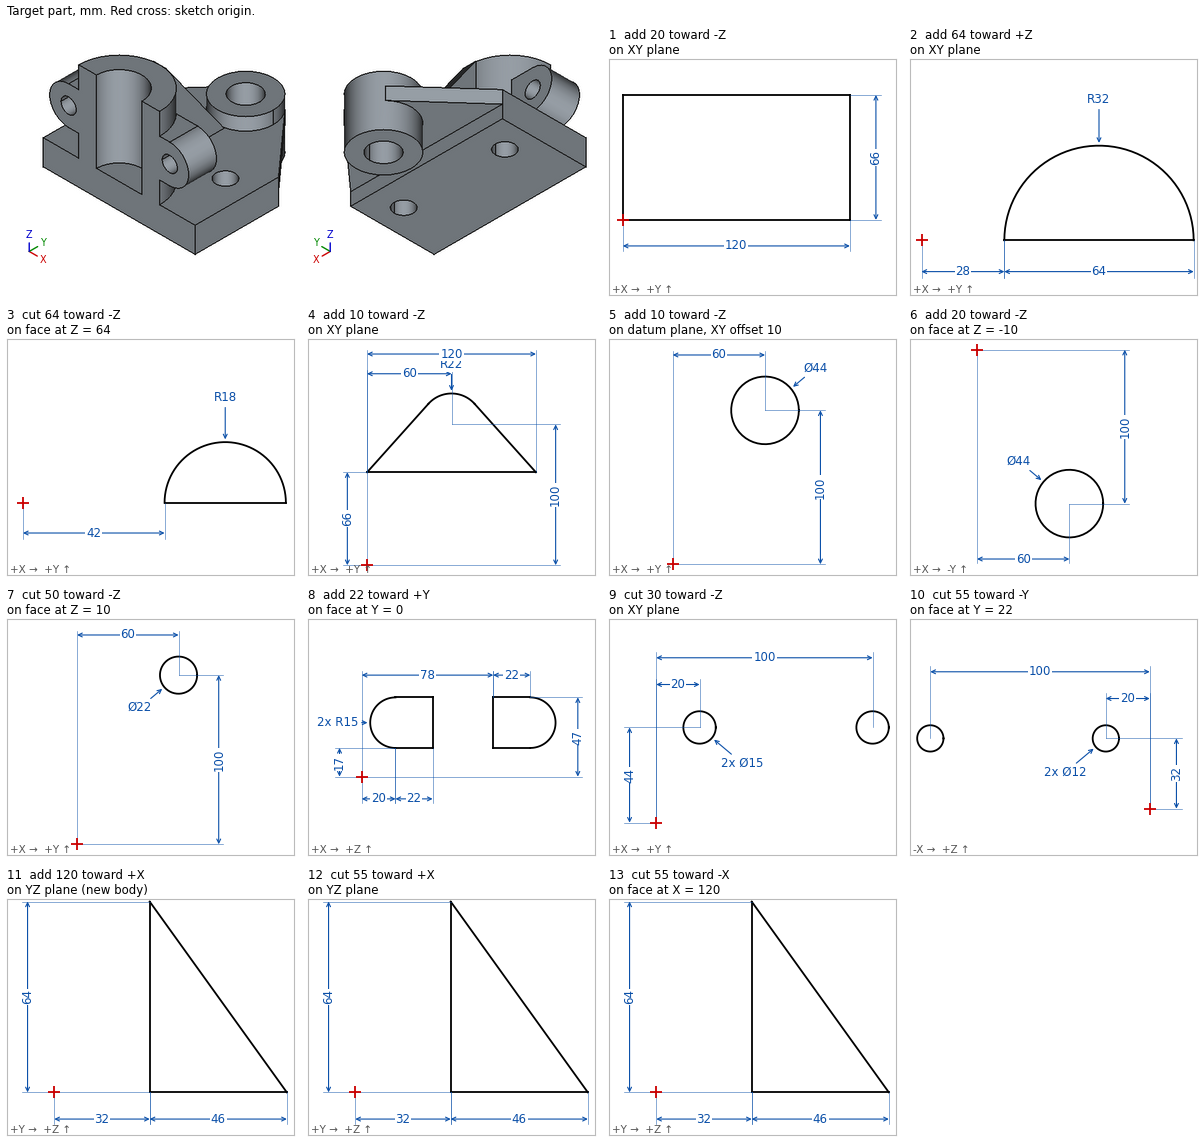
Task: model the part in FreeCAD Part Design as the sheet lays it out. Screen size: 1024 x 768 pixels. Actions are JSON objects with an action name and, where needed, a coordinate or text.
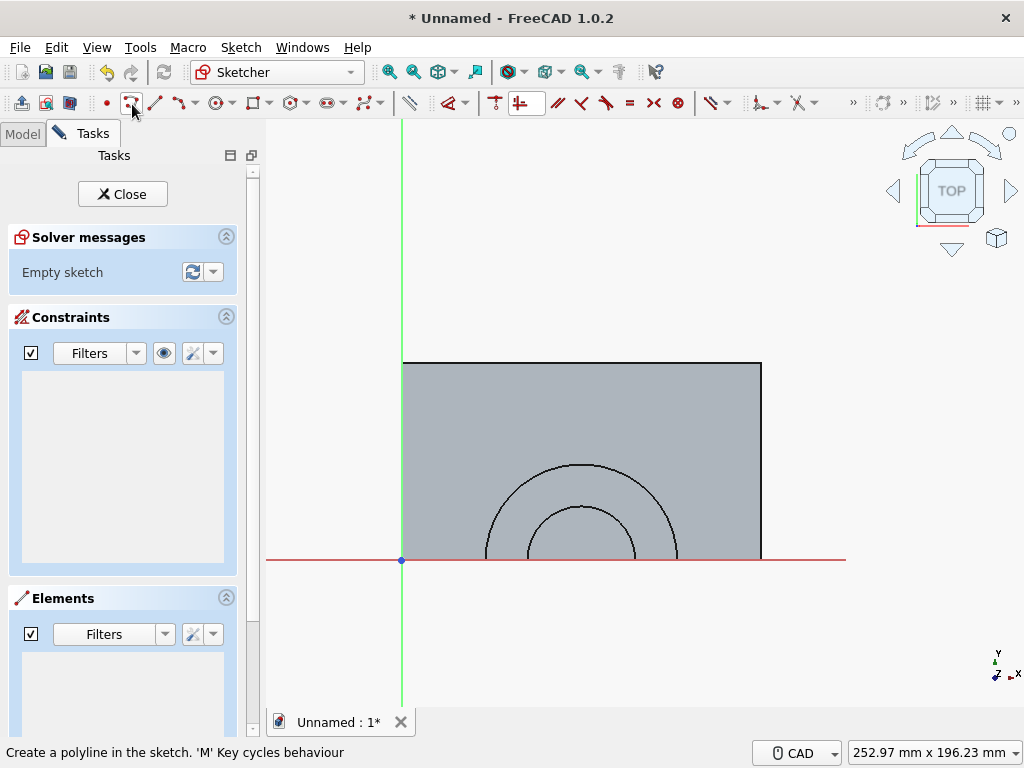
{"action": "left_click", "coordinate": [532, 217]}
{"action": "left_click", "coordinate": [402, 363]}
{"action": "left_click", "coordinate": [761, 363]}
{"action": "left_click", "coordinate": [630, 217]}
{"action": "right_click", "coordinate": [630, 217]}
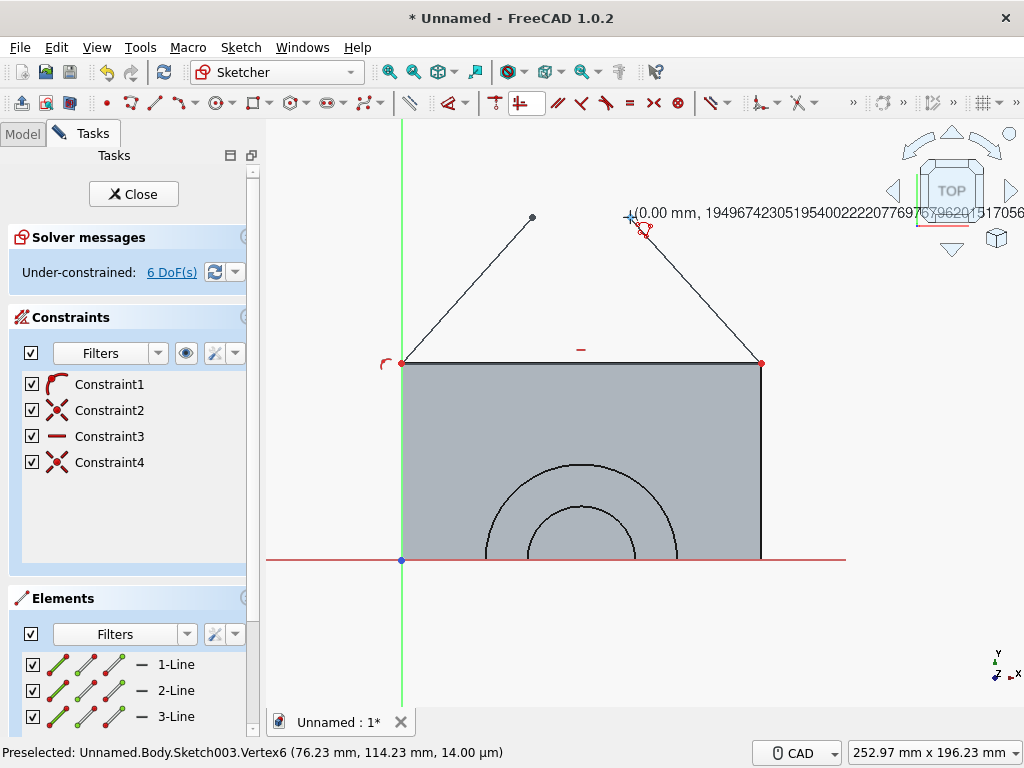
{"action": "left_click", "coordinate": [180, 104]}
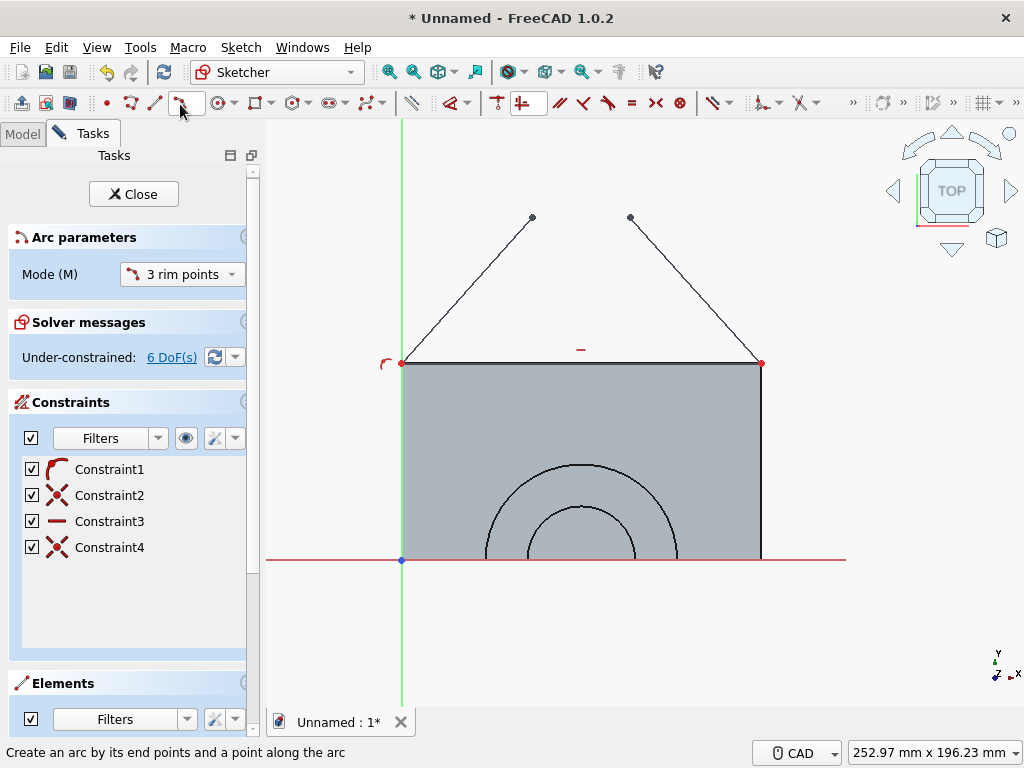
{"action": "left_click", "coordinate": [630, 218]}
{"action": "left_click", "coordinate": [532, 218]}
{"action": "left_click", "coordinate": [581, 195]}
{"action": "key", "text": "Escape"}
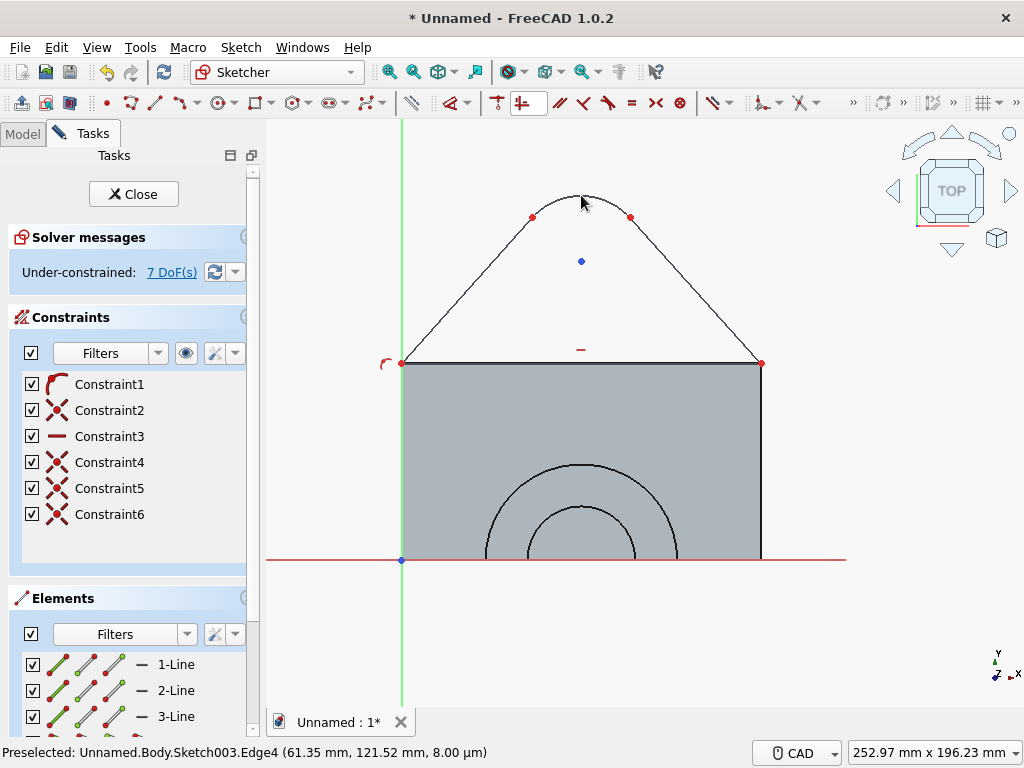
{"action": "left_click", "coordinate": [493, 262]}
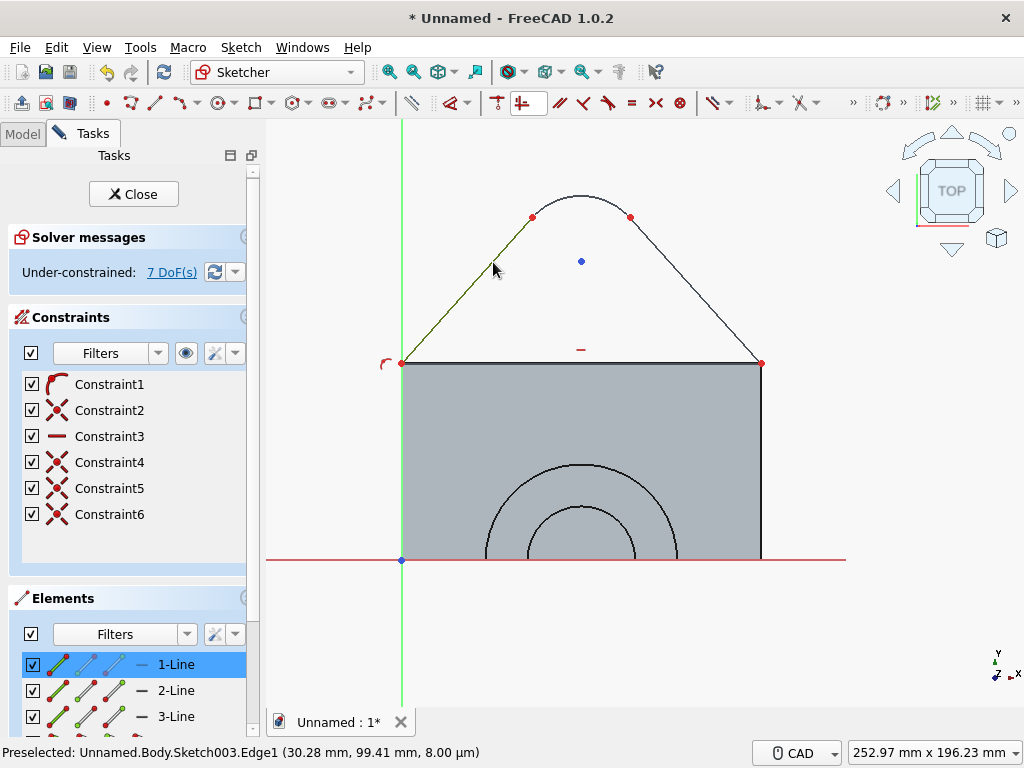
{"action": "left_click", "coordinate": [603, 200]}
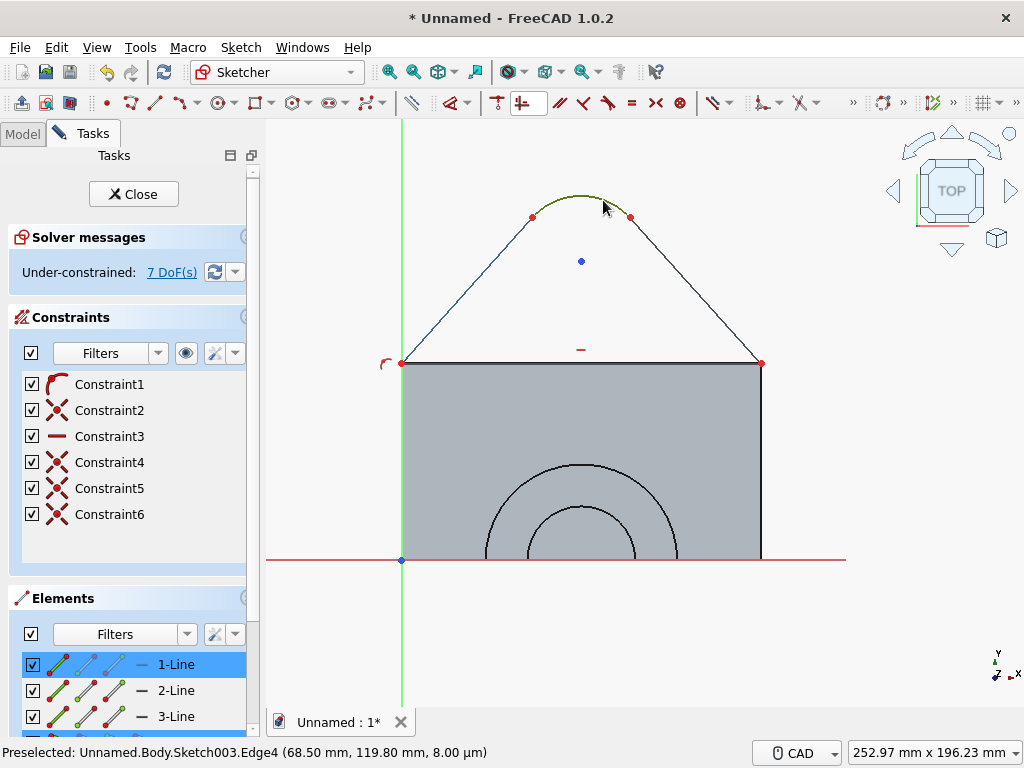
{"action": "left_click", "coordinate": [608, 104]}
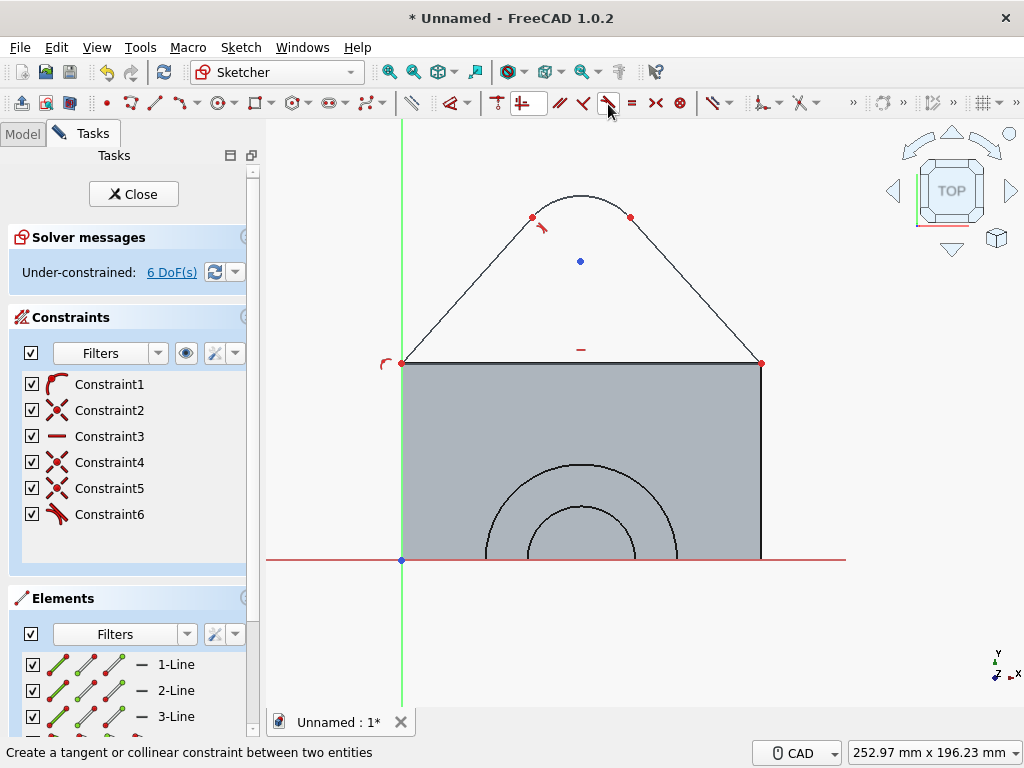
{"action": "left_click", "coordinate": [722, 320]}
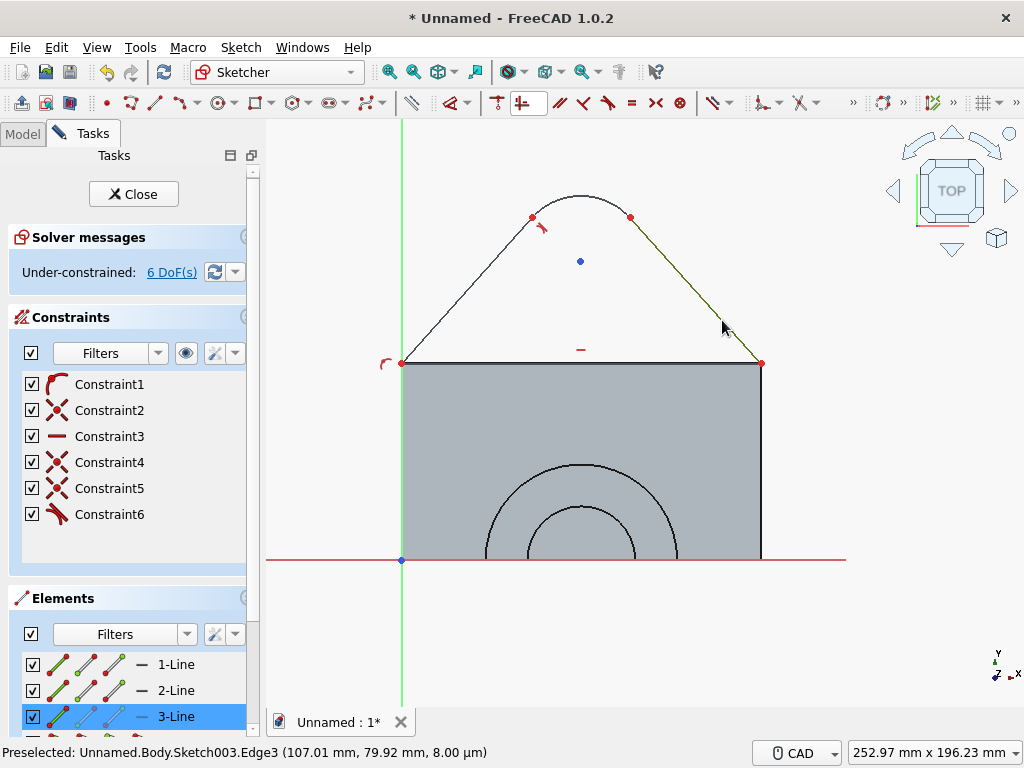
{"action": "left_click", "coordinate": [603, 200]}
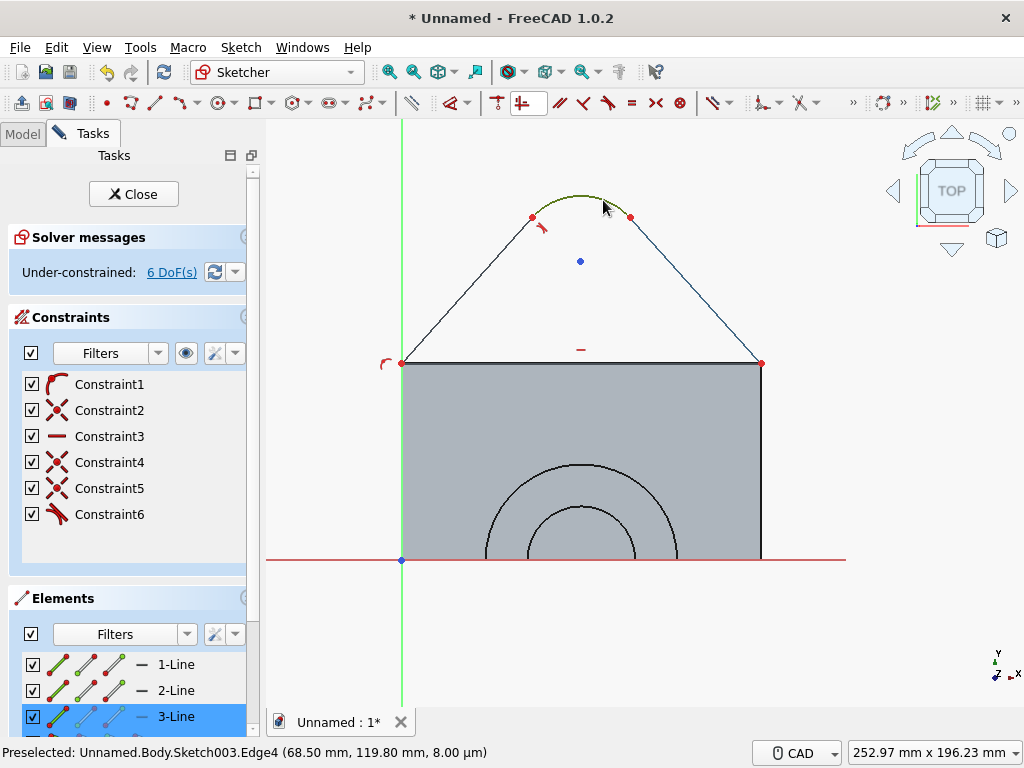
{"action": "left_click", "coordinate": [608, 104]}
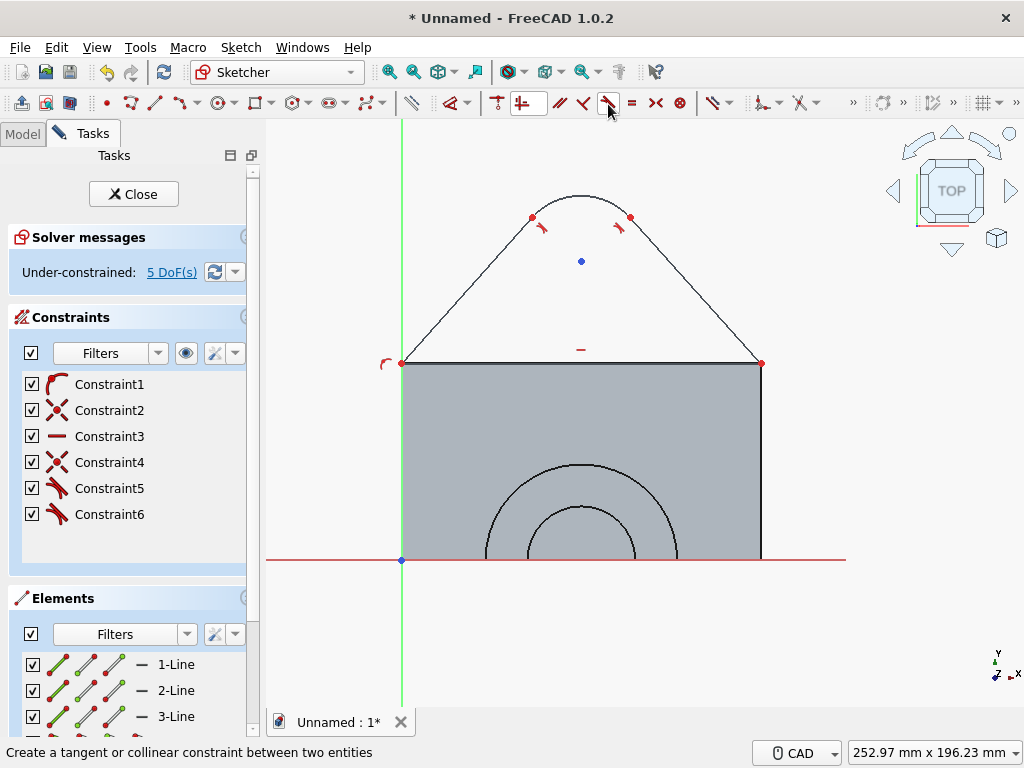
{"action": "left_click", "coordinate": [450, 104]}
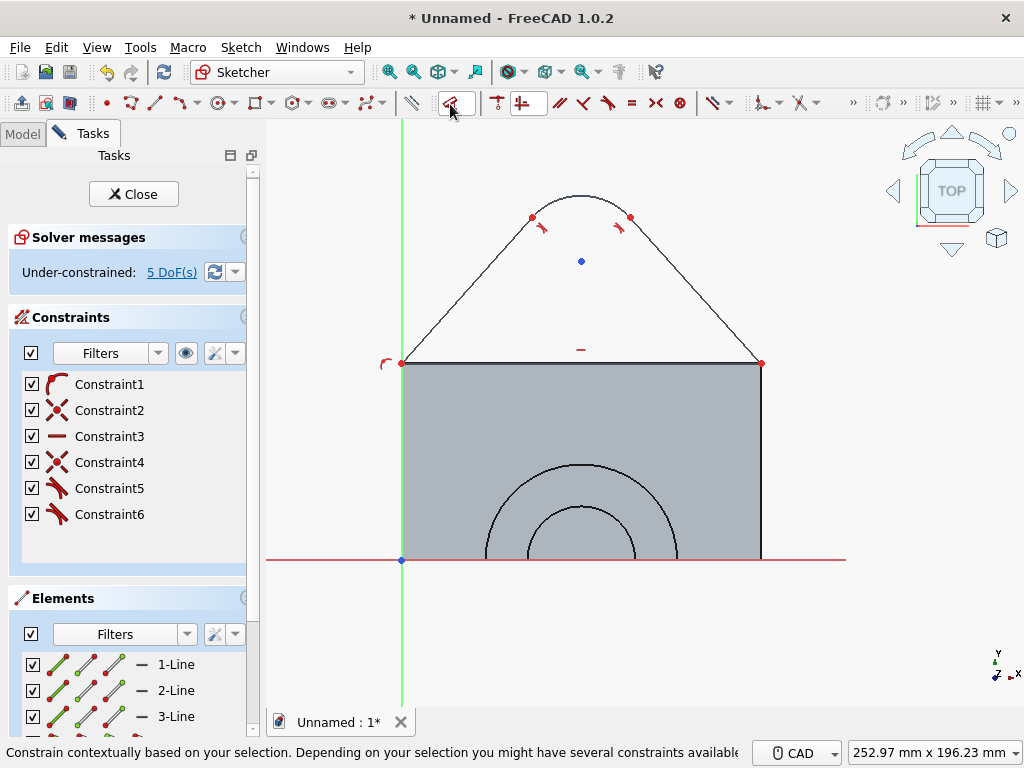
{"action": "left_click", "coordinate": [603, 200]}
{"action": "left_click", "coordinate": [614, 170]}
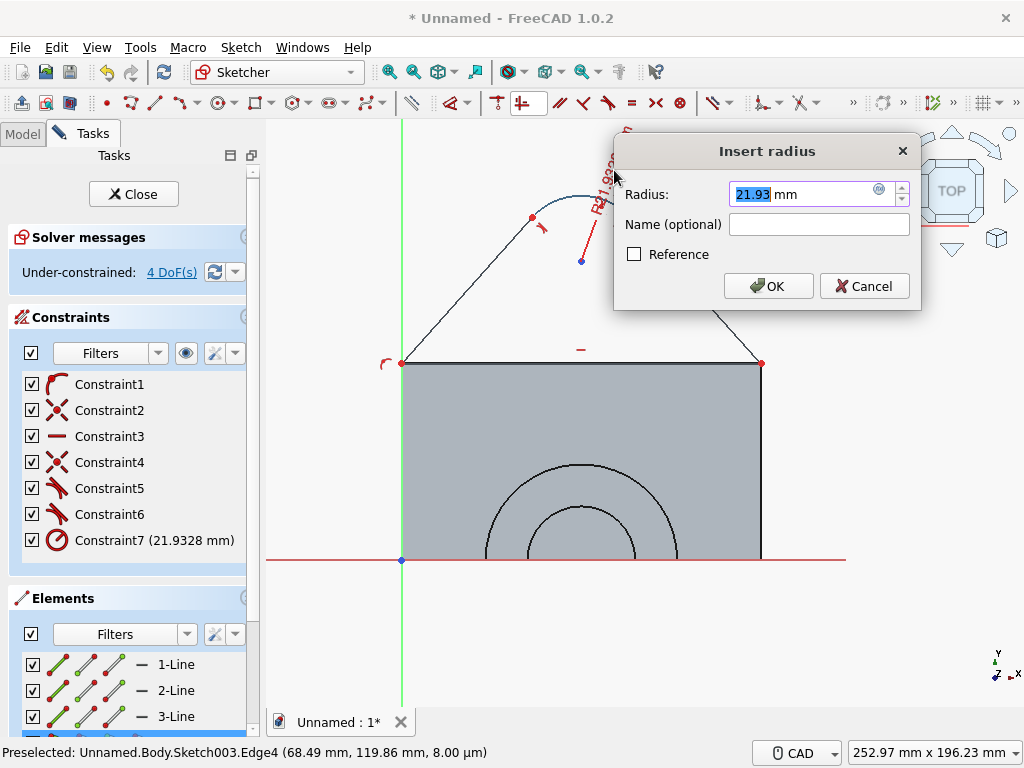
{"action": "type", "text": "22"}
{"action": "key", "text": "Return"}